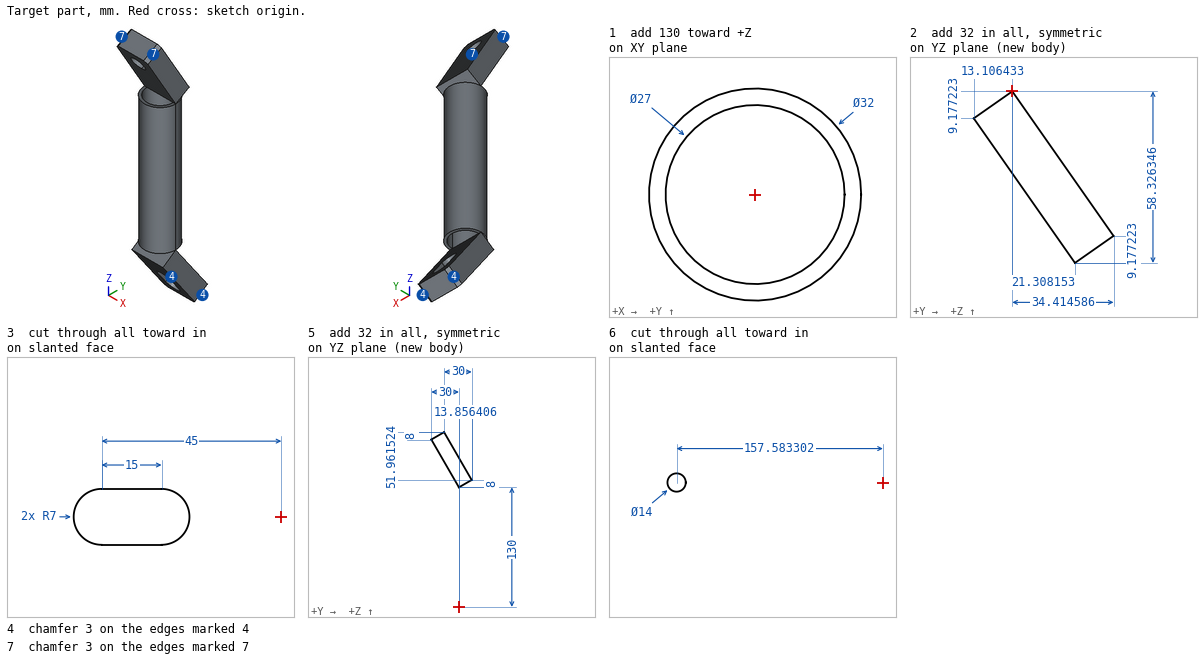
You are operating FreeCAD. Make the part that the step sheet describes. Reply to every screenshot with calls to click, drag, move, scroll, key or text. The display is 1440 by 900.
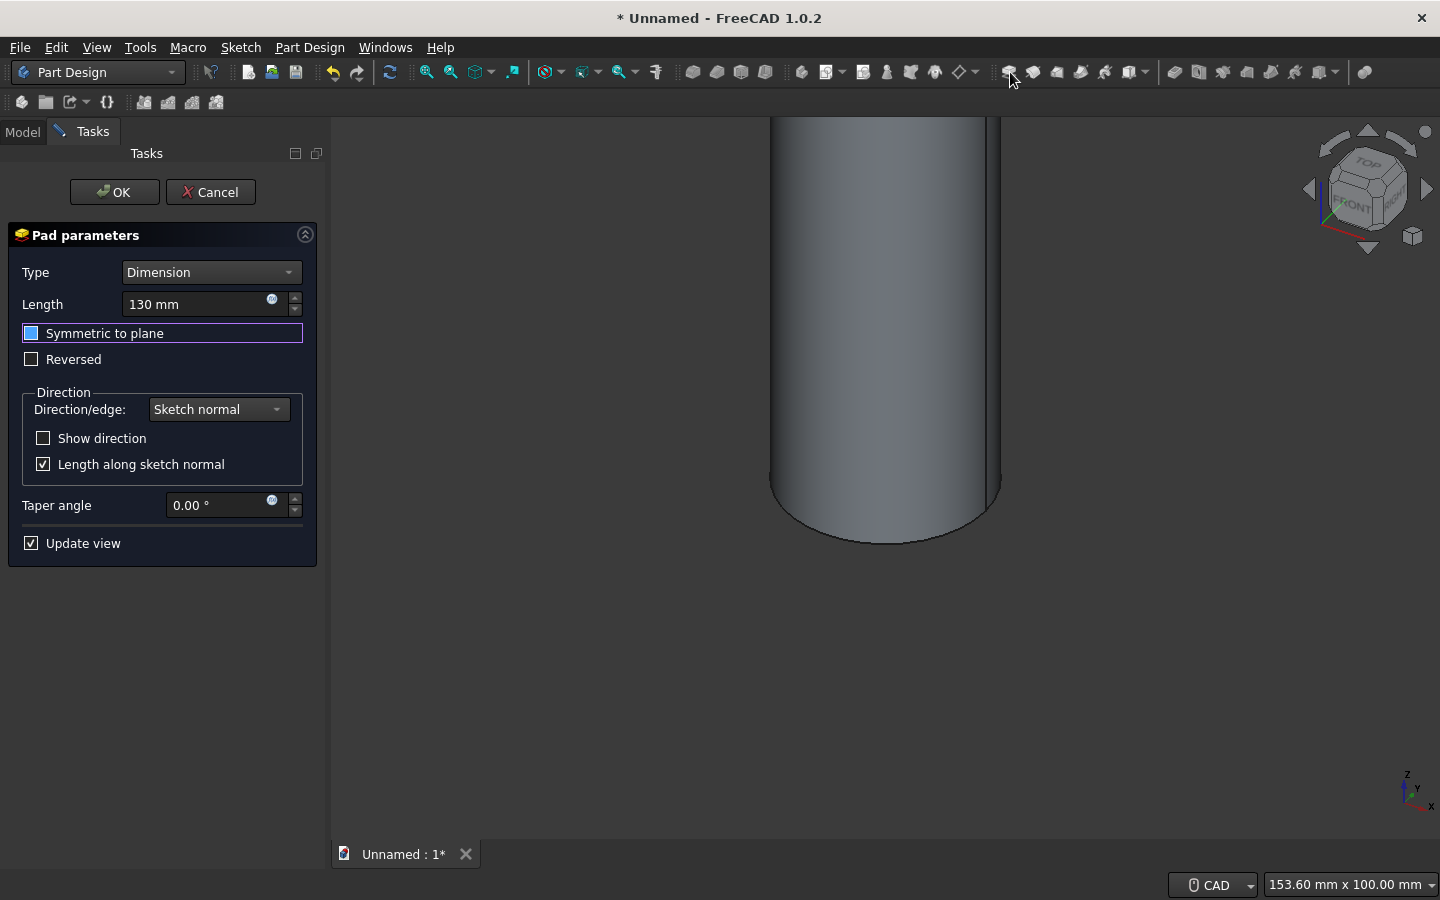
click(115, 192)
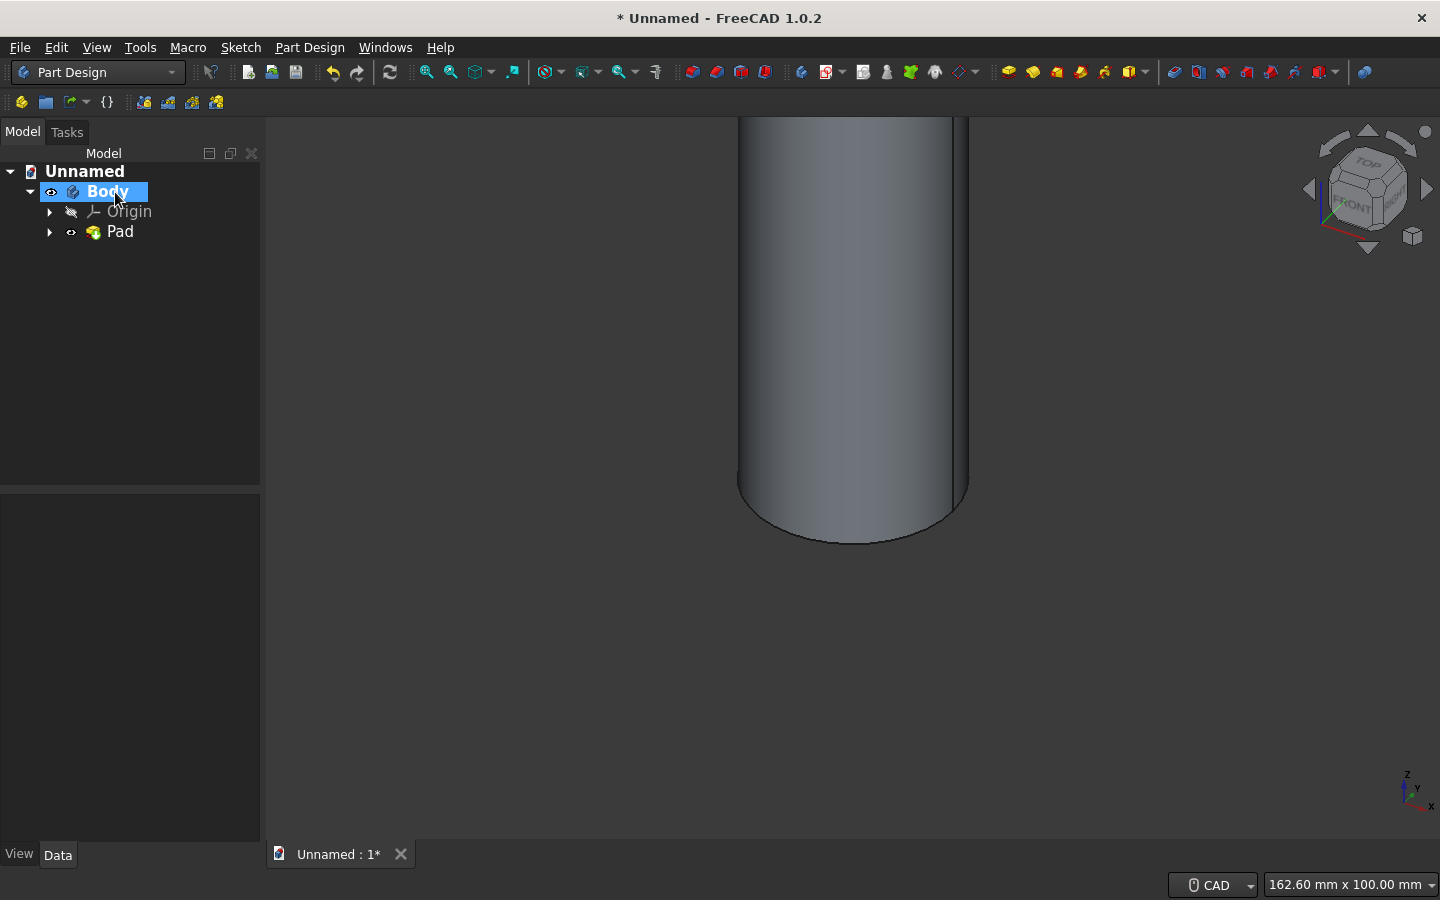
key(v)
key(f)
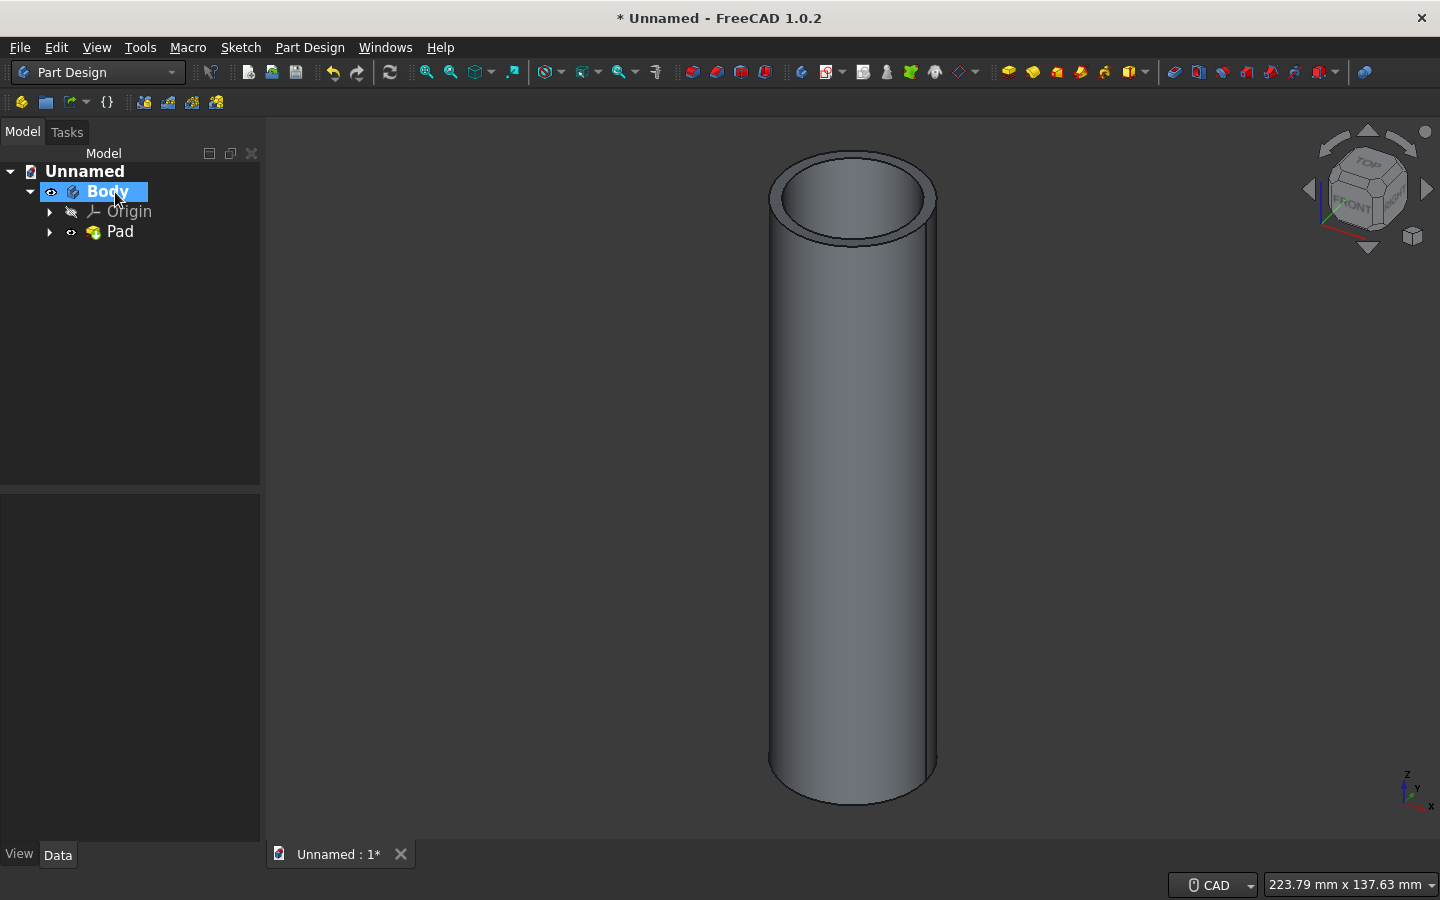
click(802, 72)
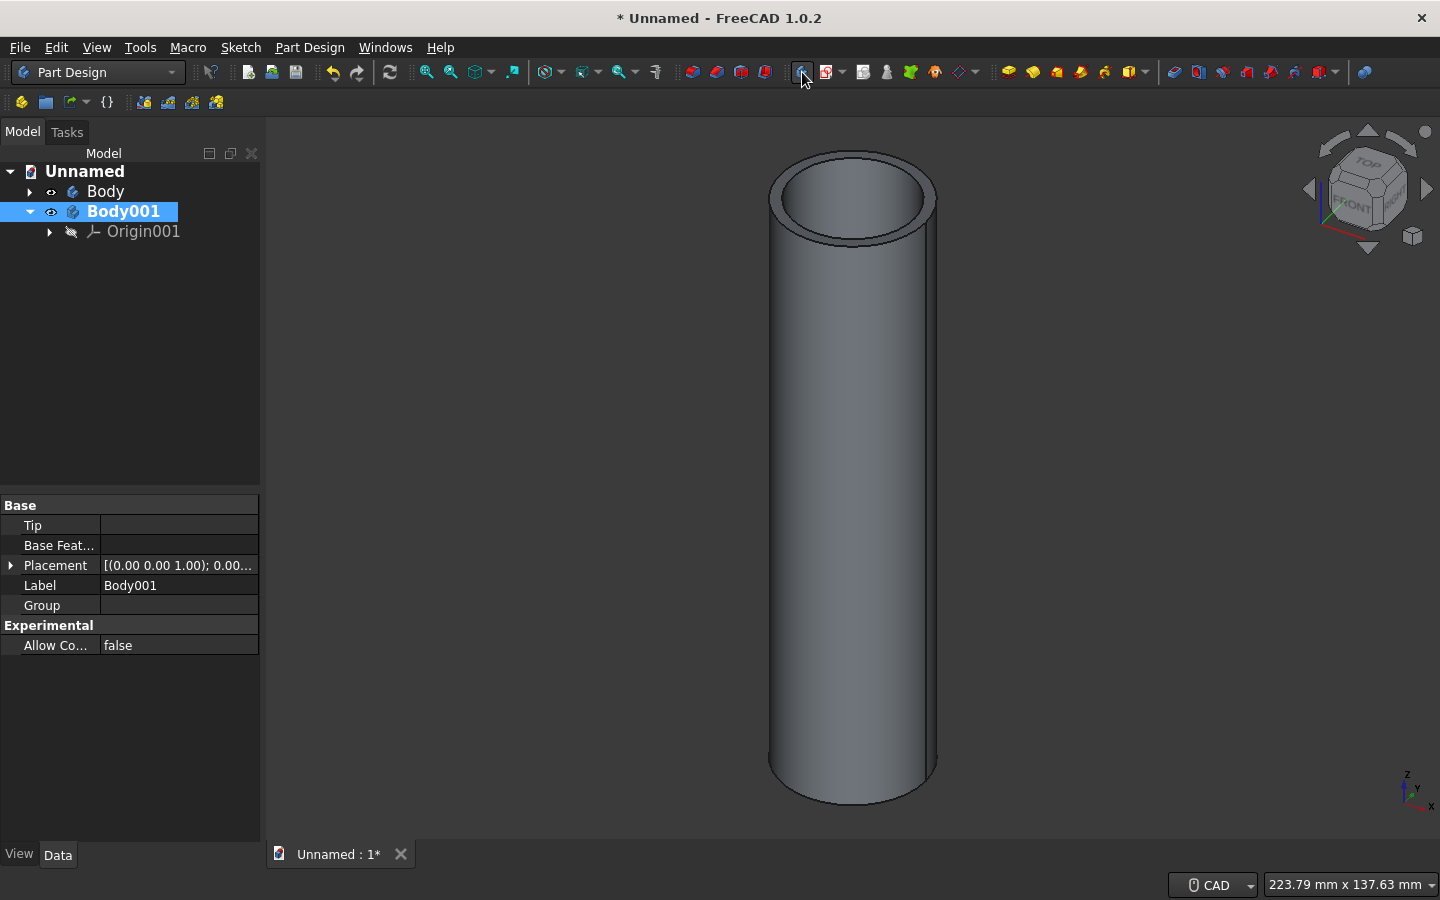
click(306, 799)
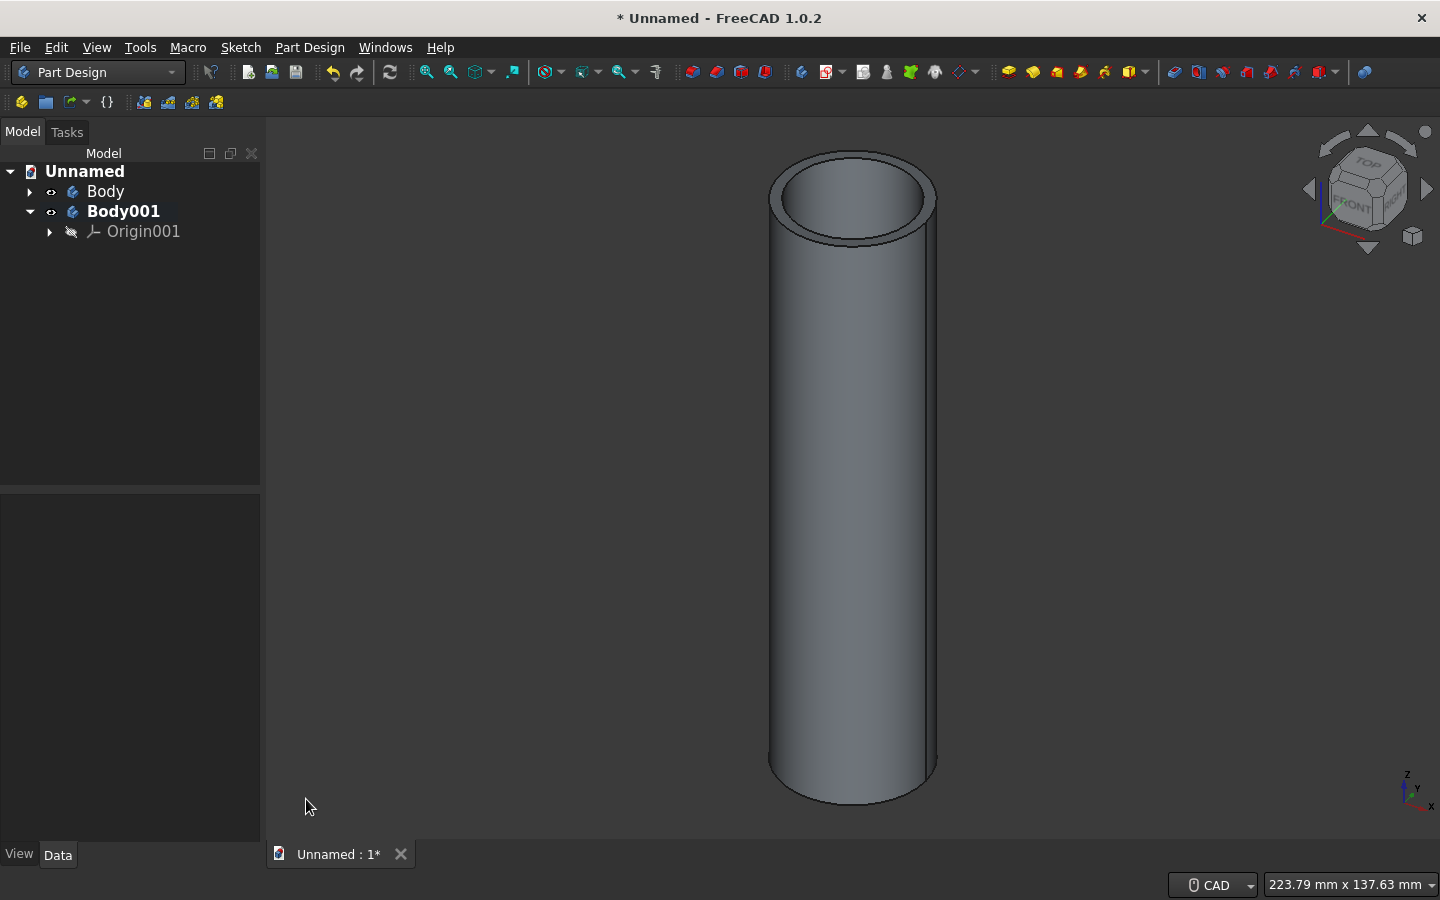
click(826, 72)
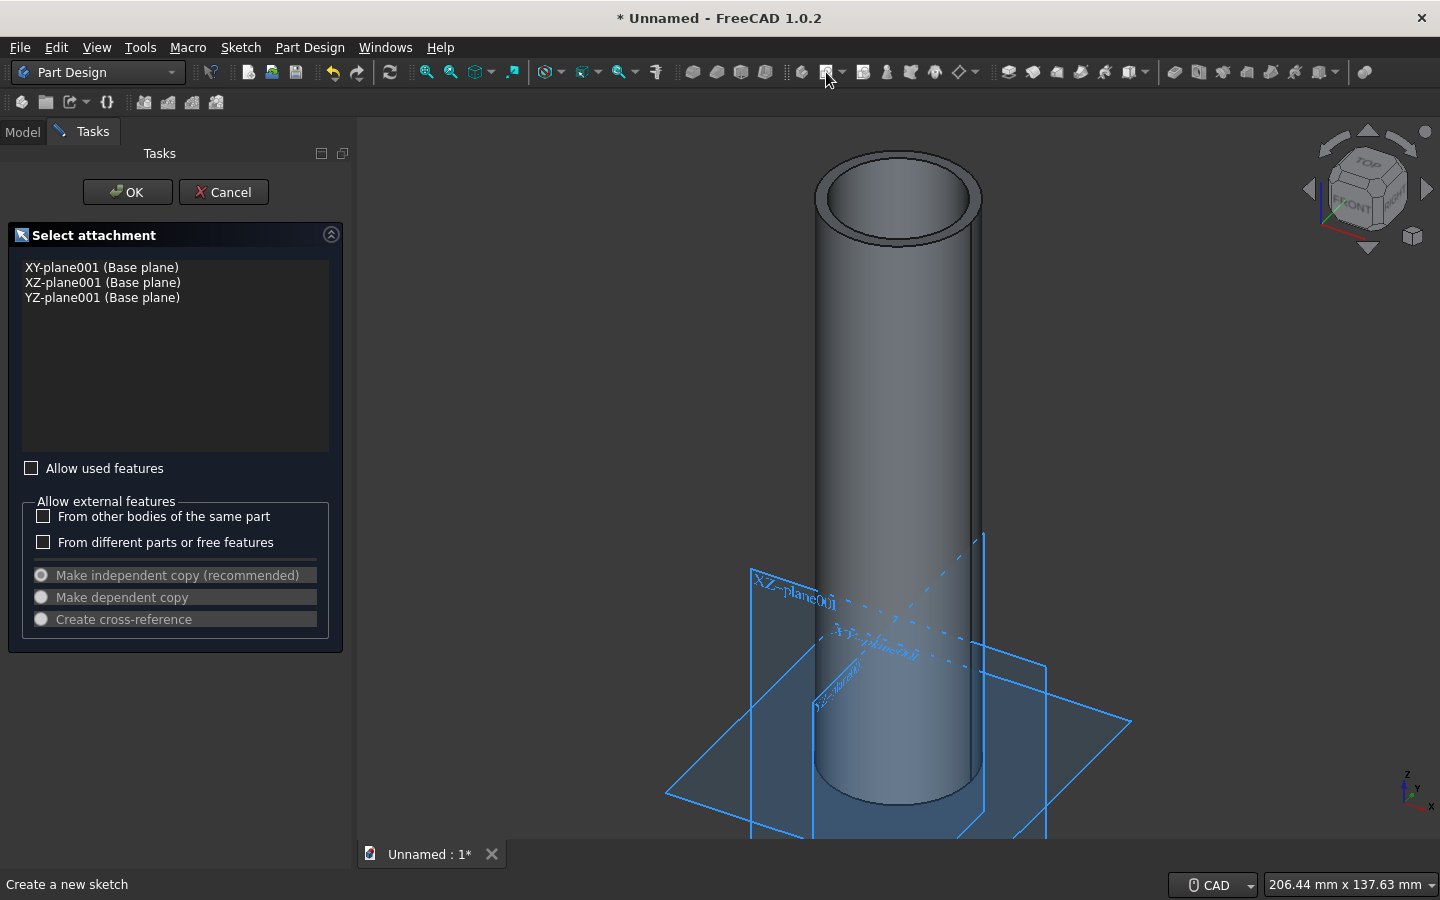
click(82, 298)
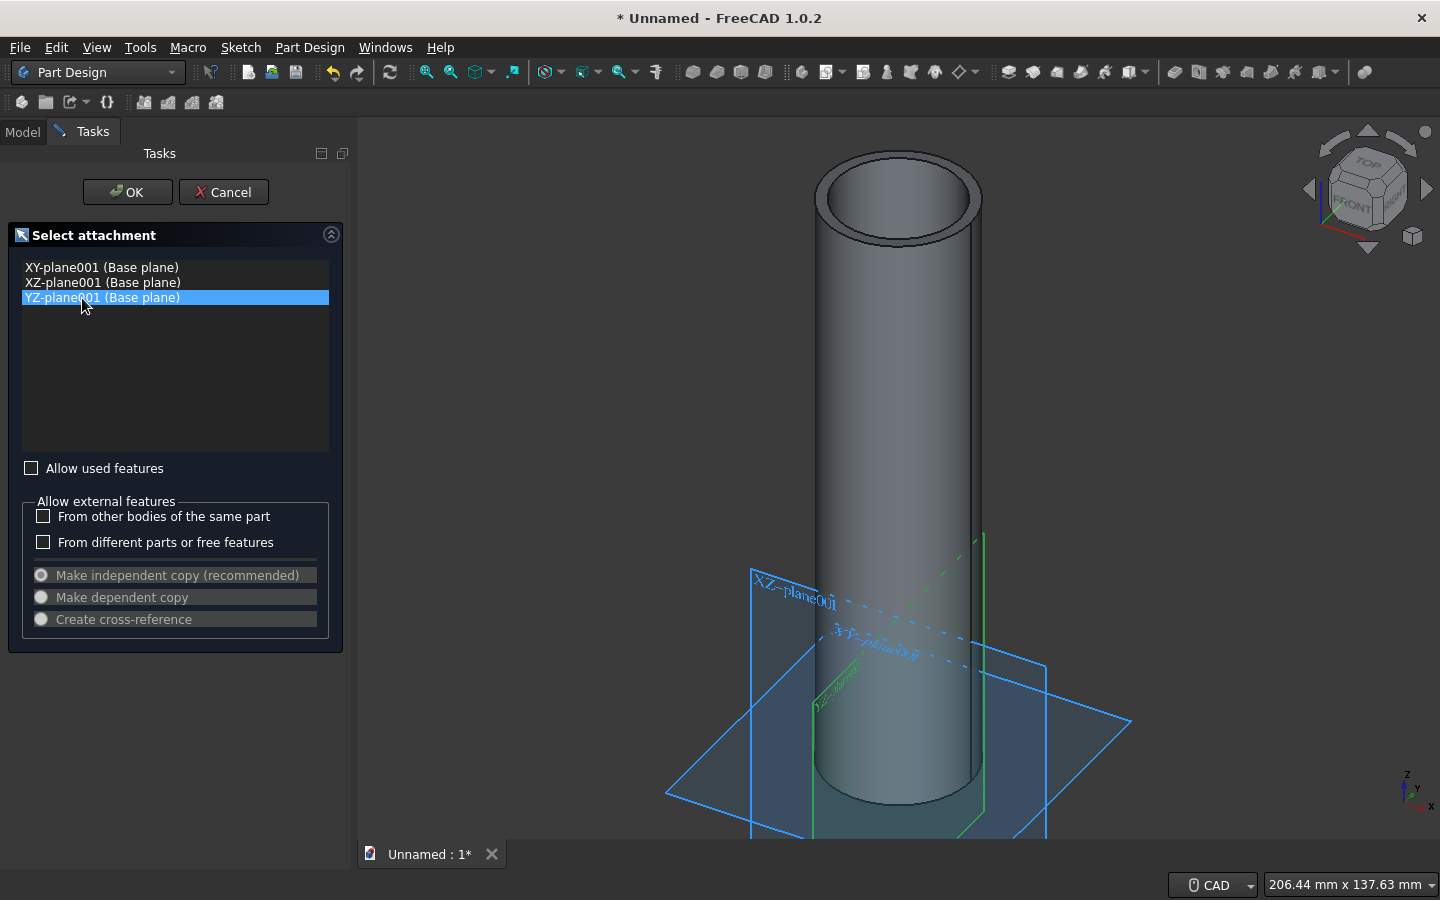
click(128, 192)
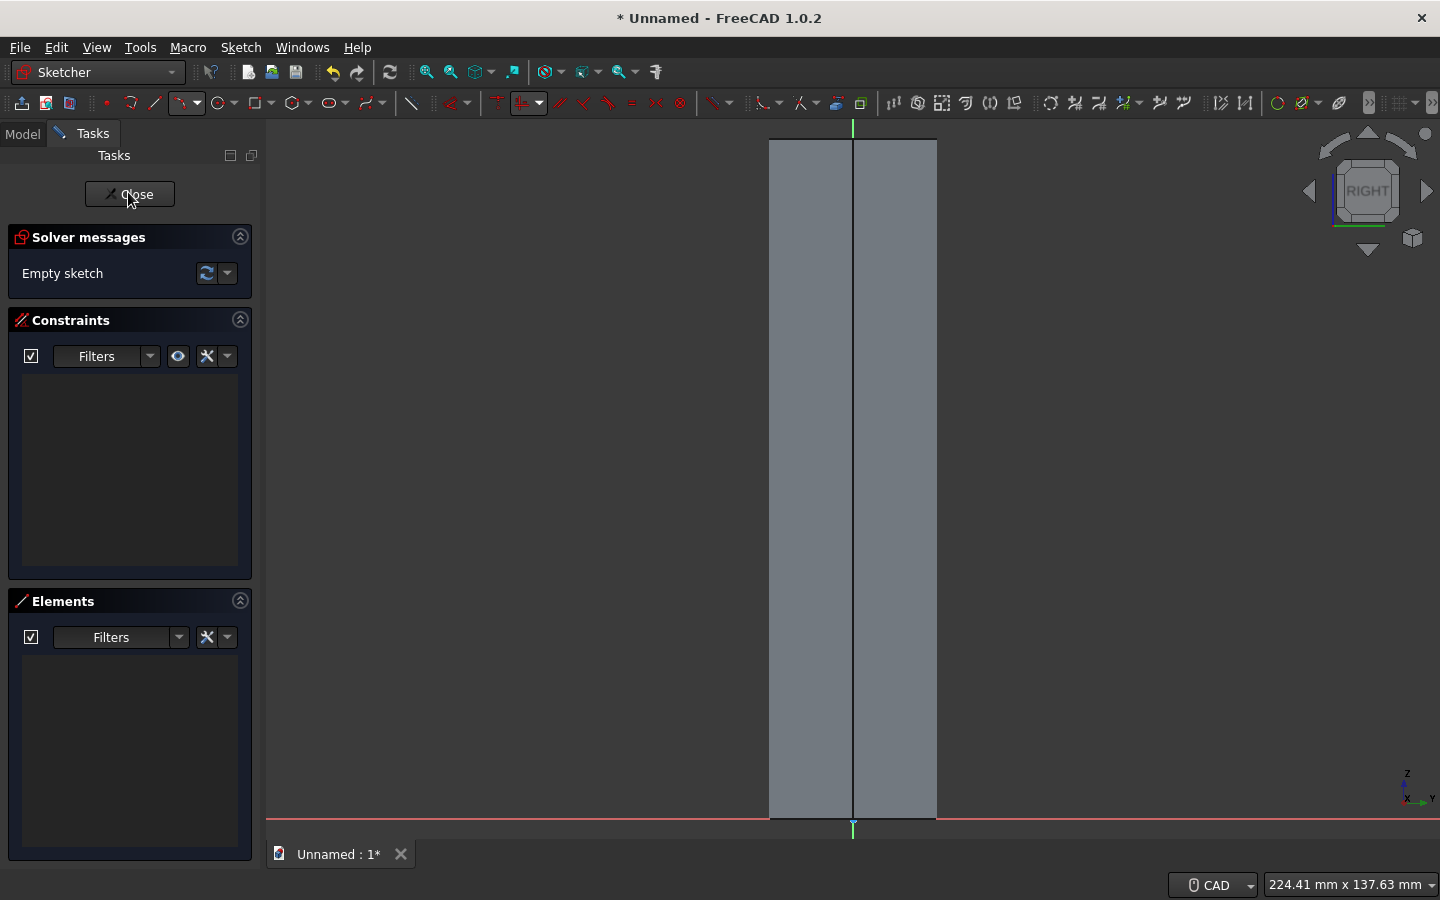
scroll(784, 479, down, 5)